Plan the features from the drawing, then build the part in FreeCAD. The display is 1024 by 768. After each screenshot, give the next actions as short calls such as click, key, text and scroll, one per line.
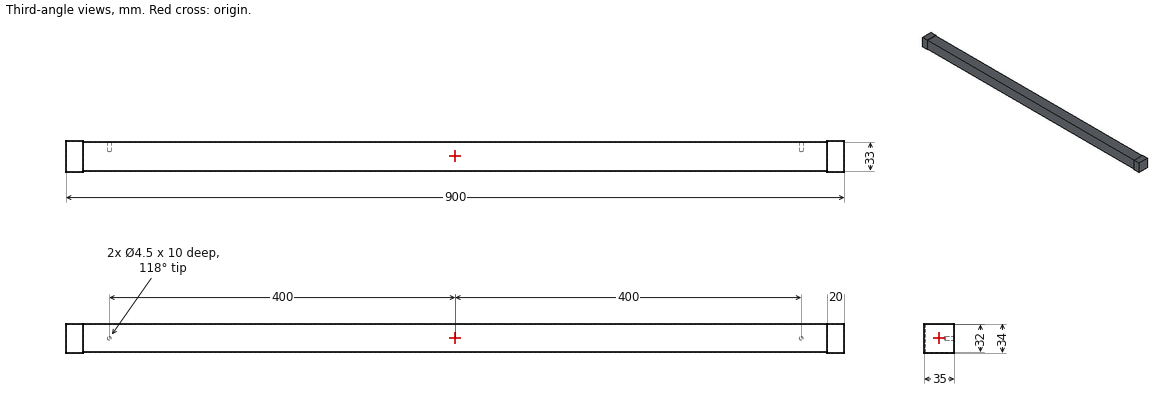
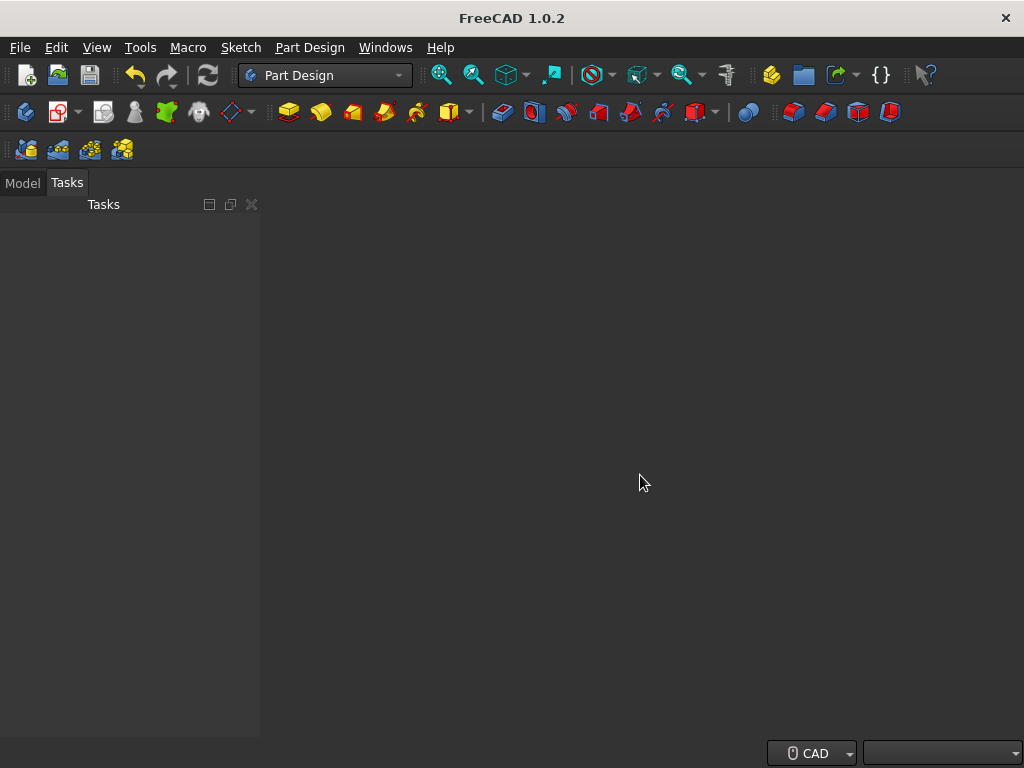
click(26, 76)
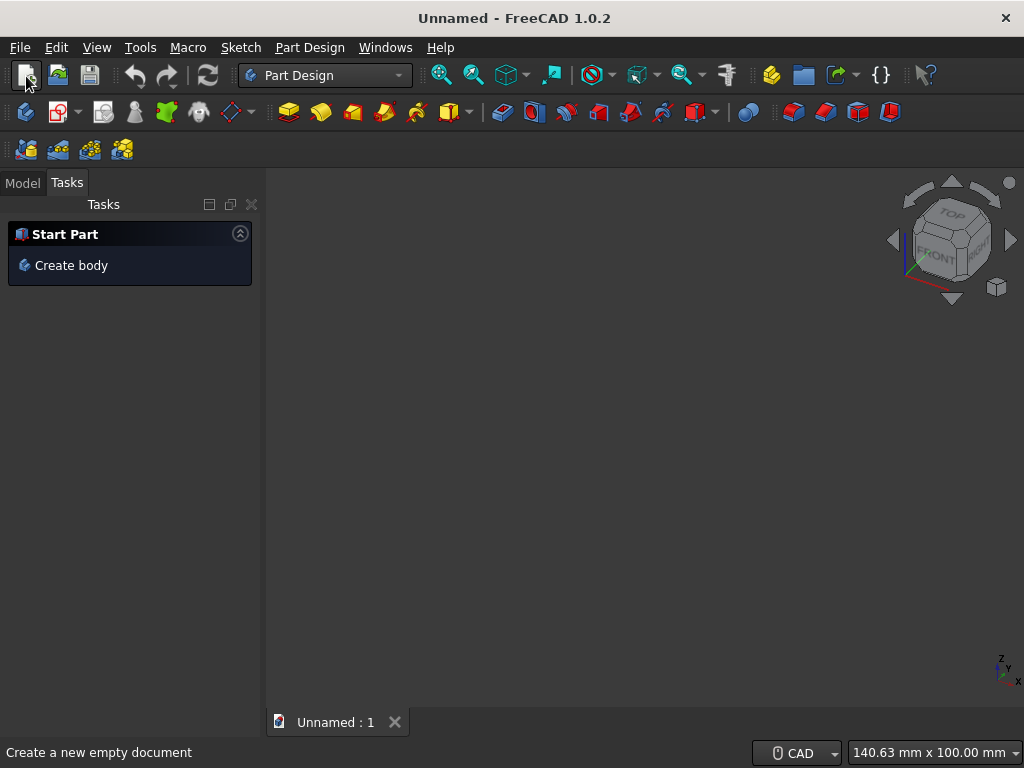
click(58, 112)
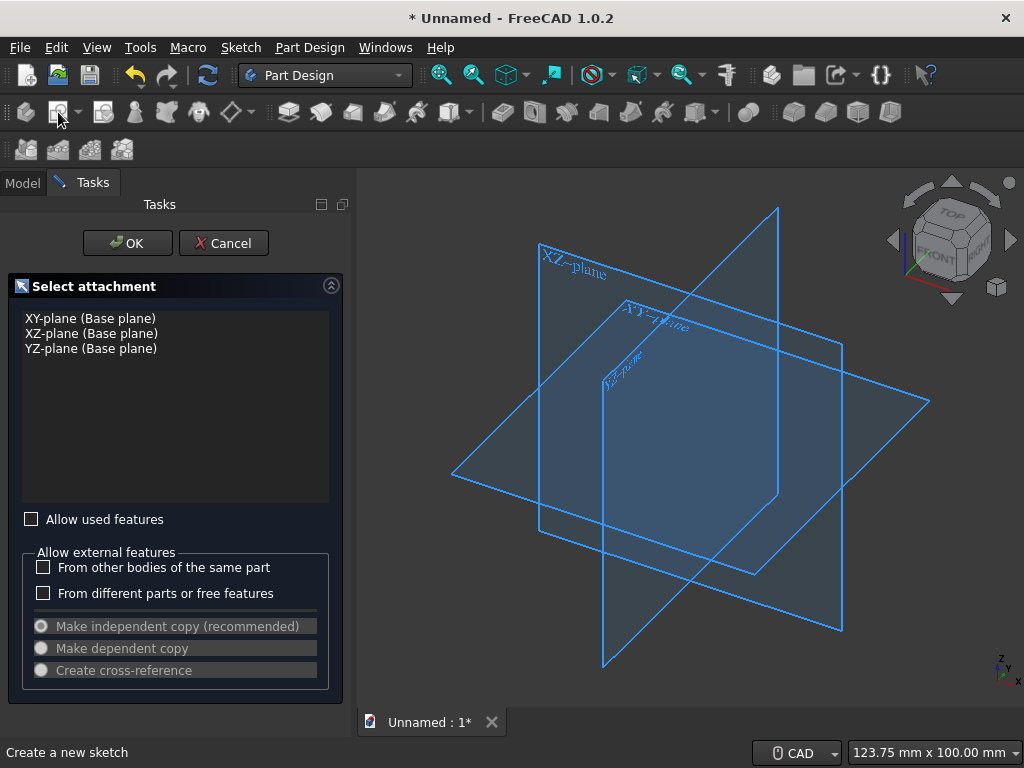
click(82, 318)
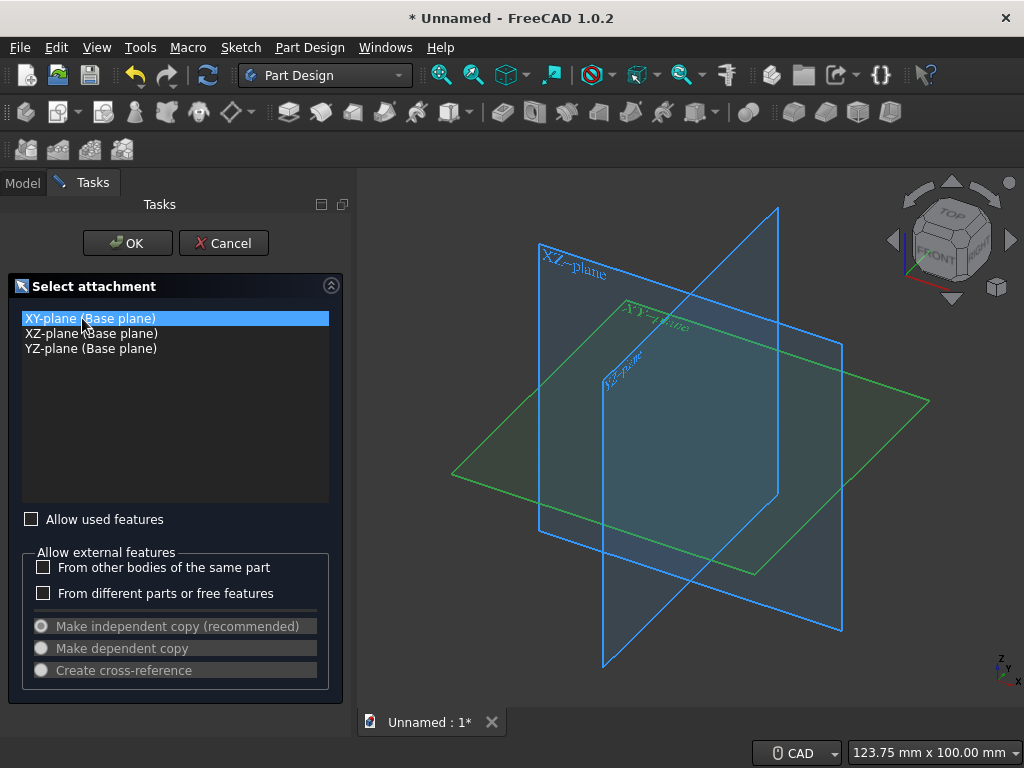
click(128, 243)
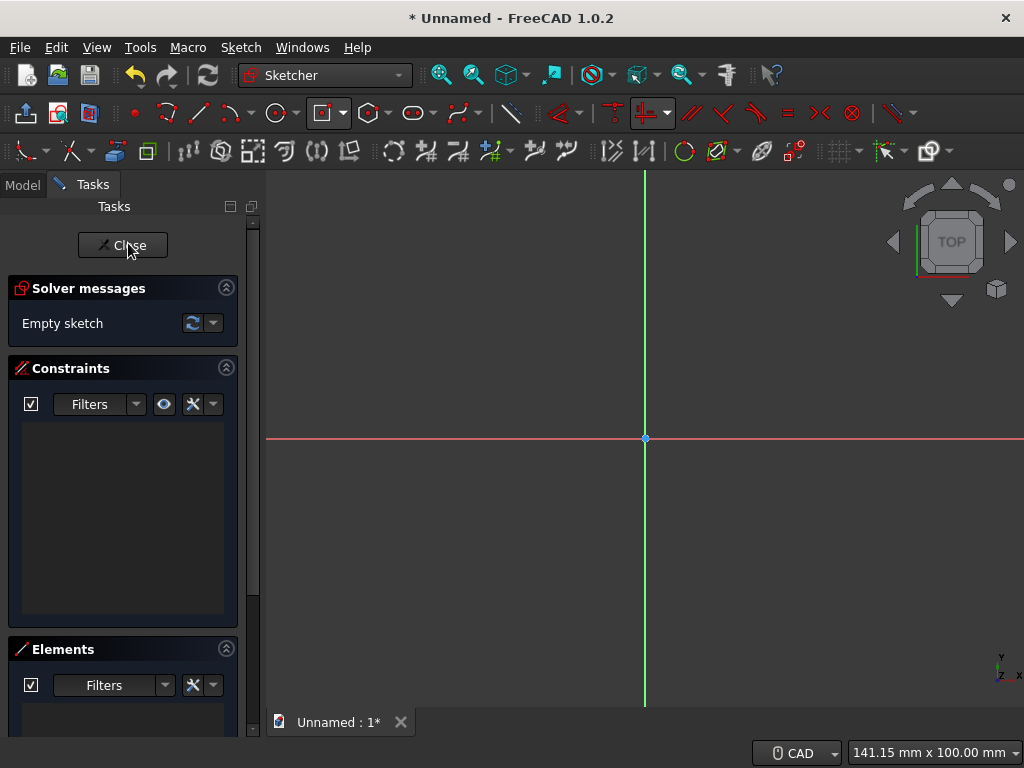
scroll(570, 438, down, 12)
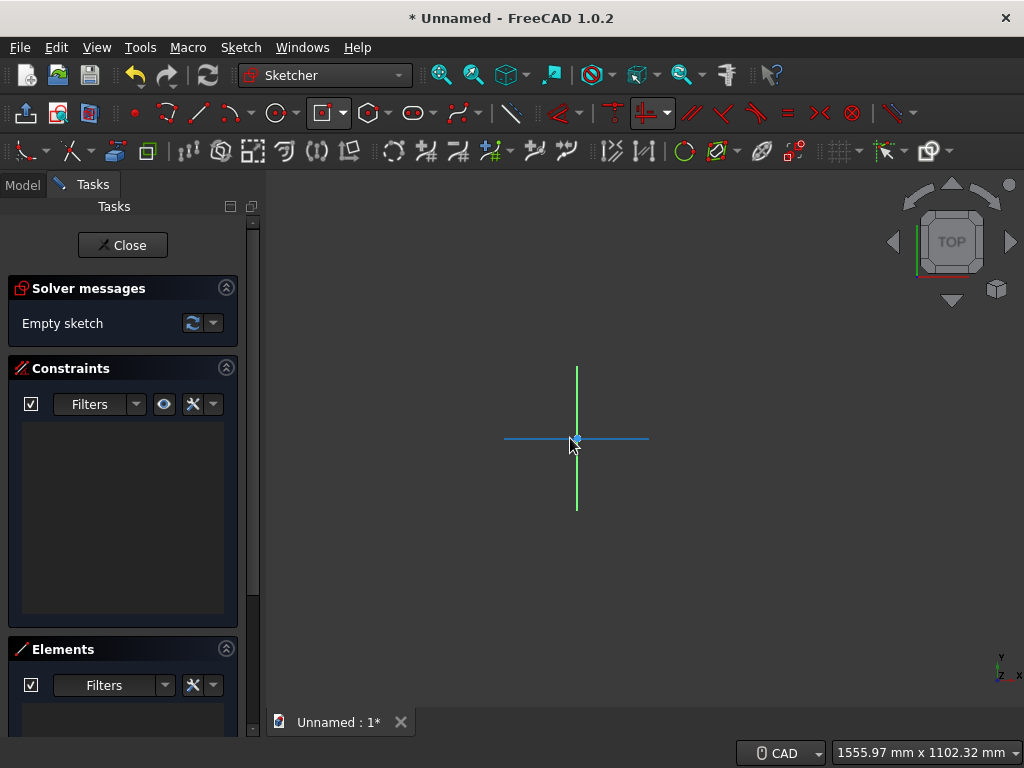
key(g)
key(v)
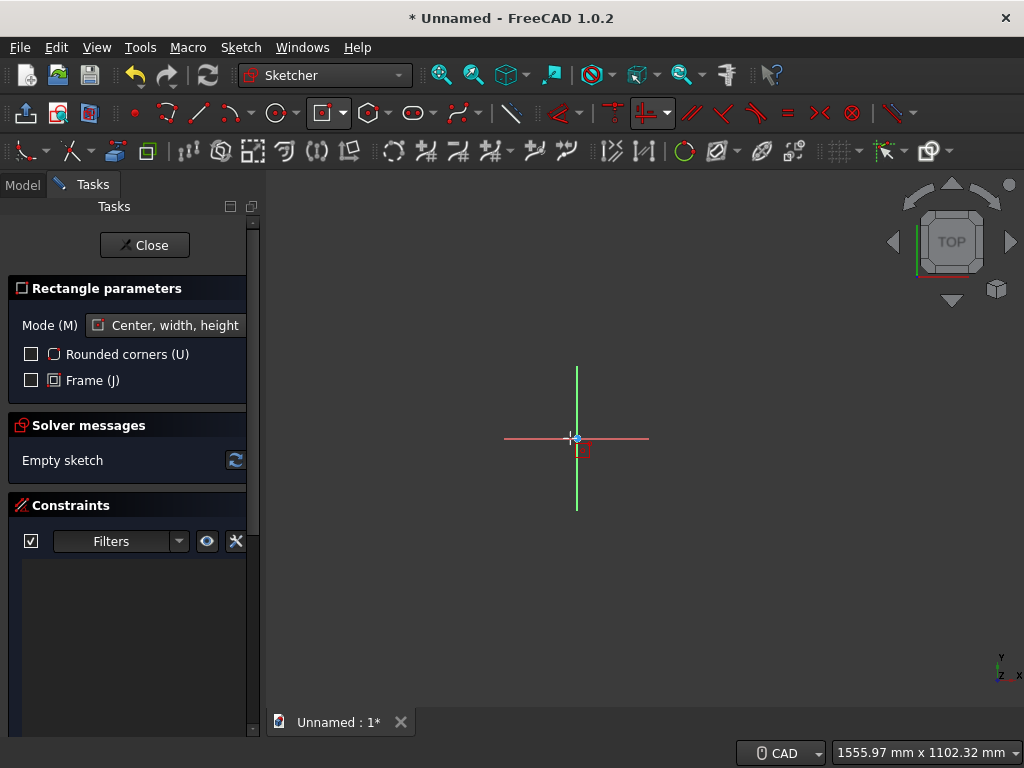
scroll(577, 438, up, 4)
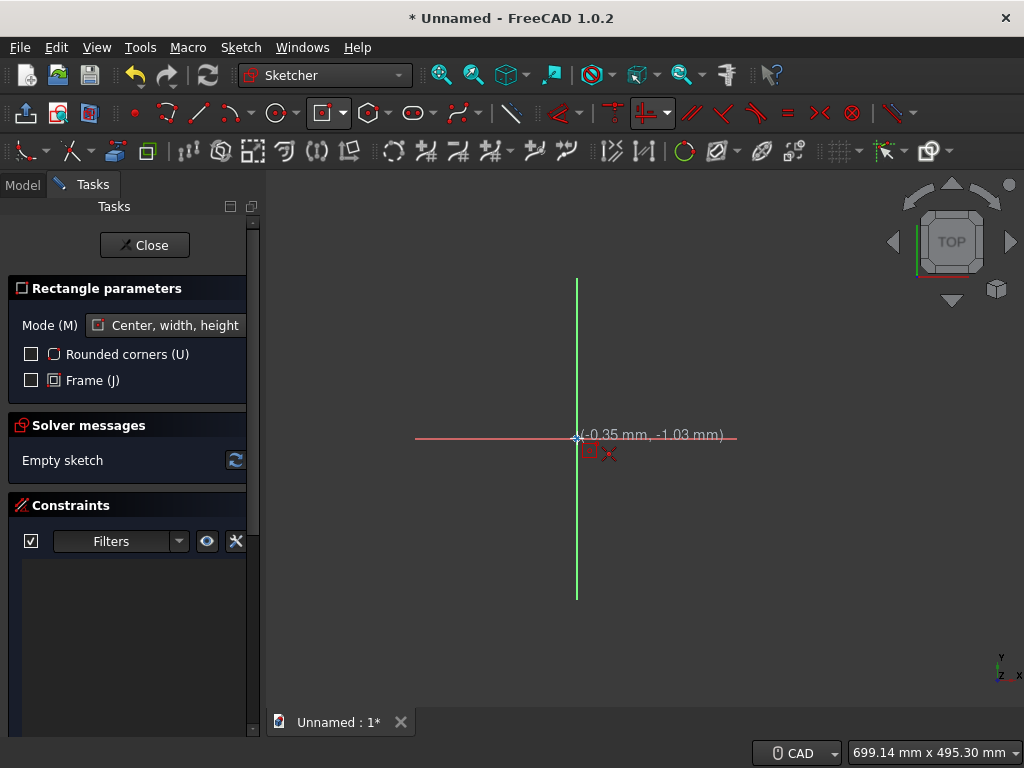
click(577, 438)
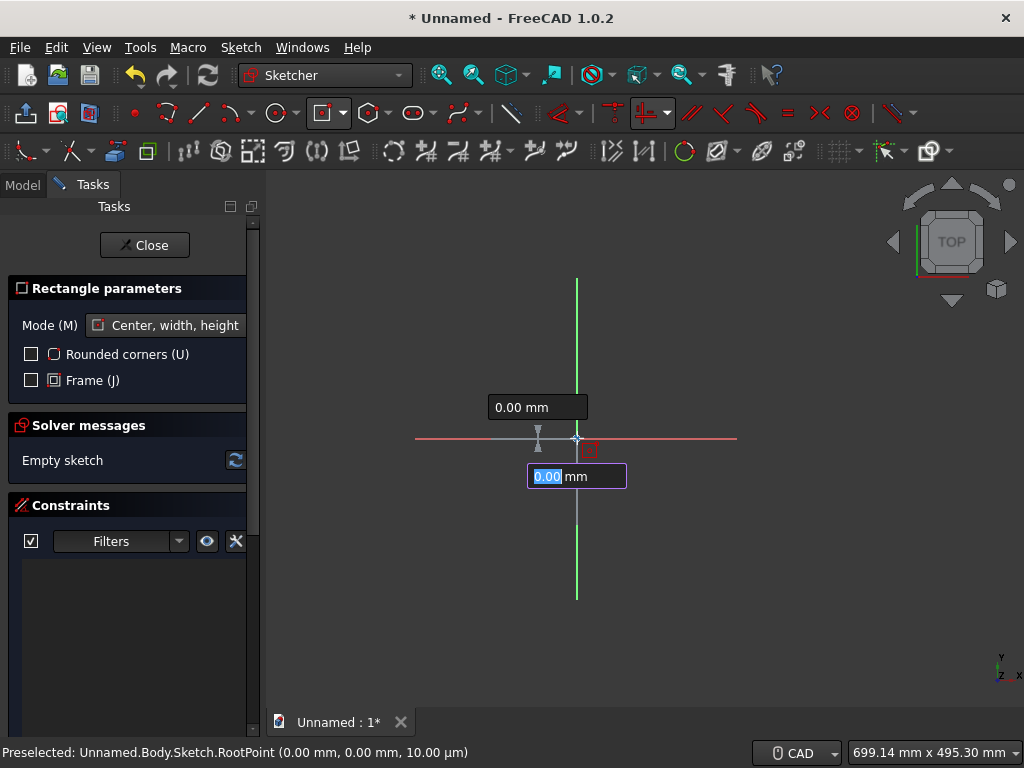
scroll(576, 438, down, 4)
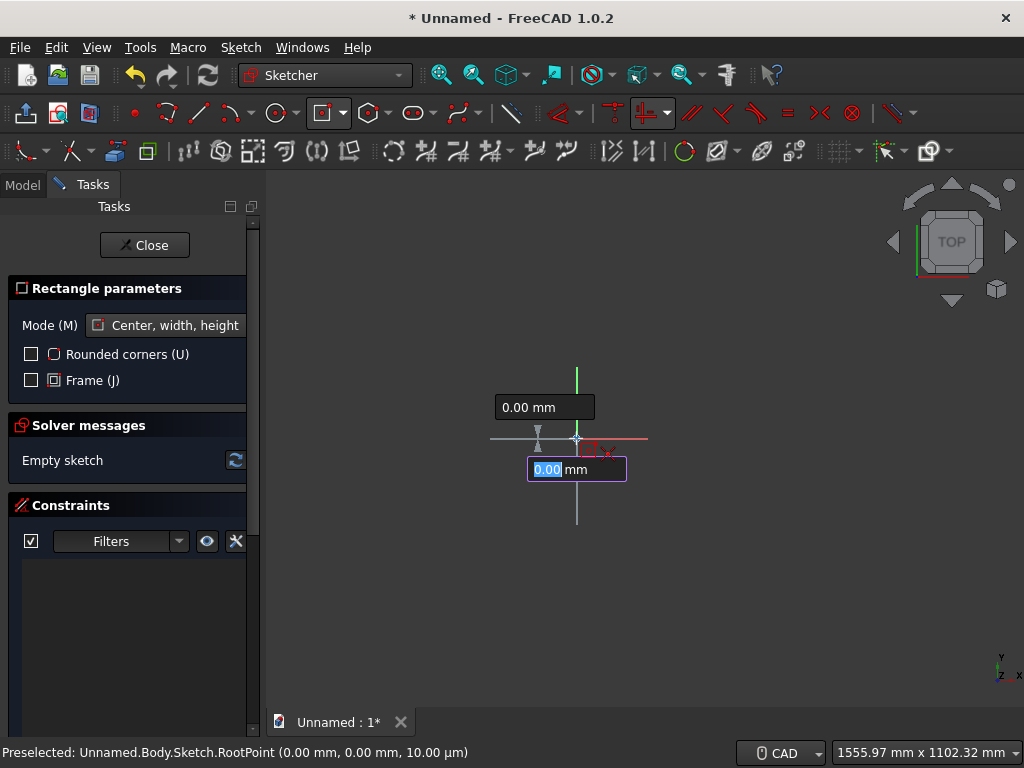
scroll(796, 430, up, 4)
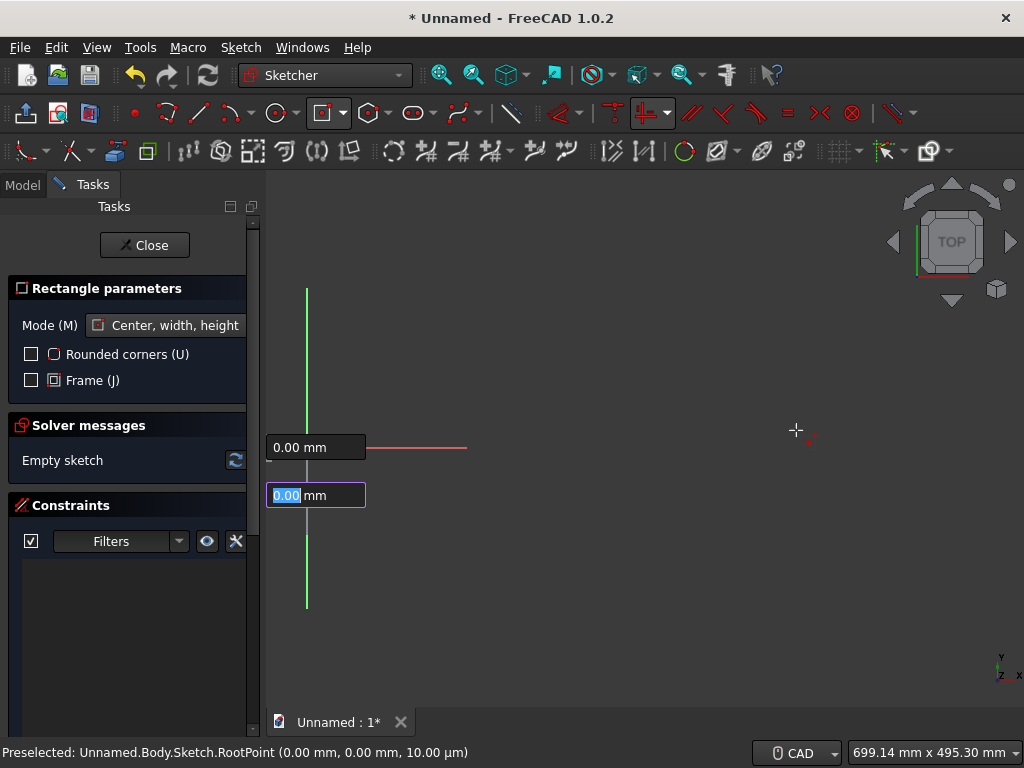
click(795, 430)
key(Escape)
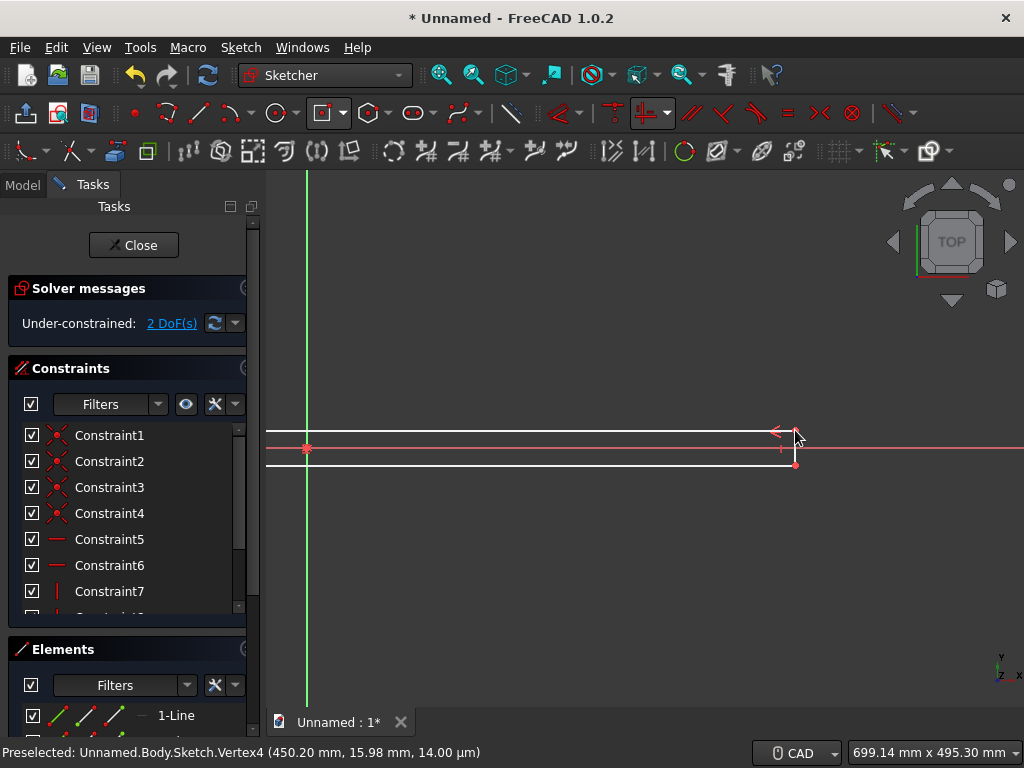
click(795, 452)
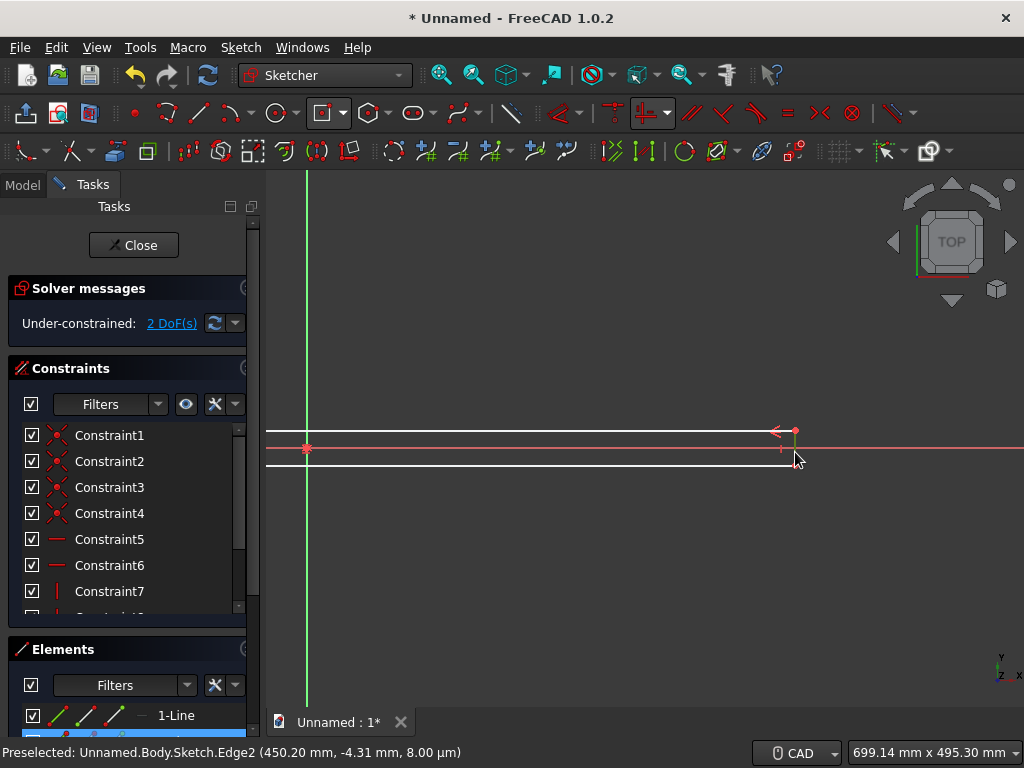
key(i)